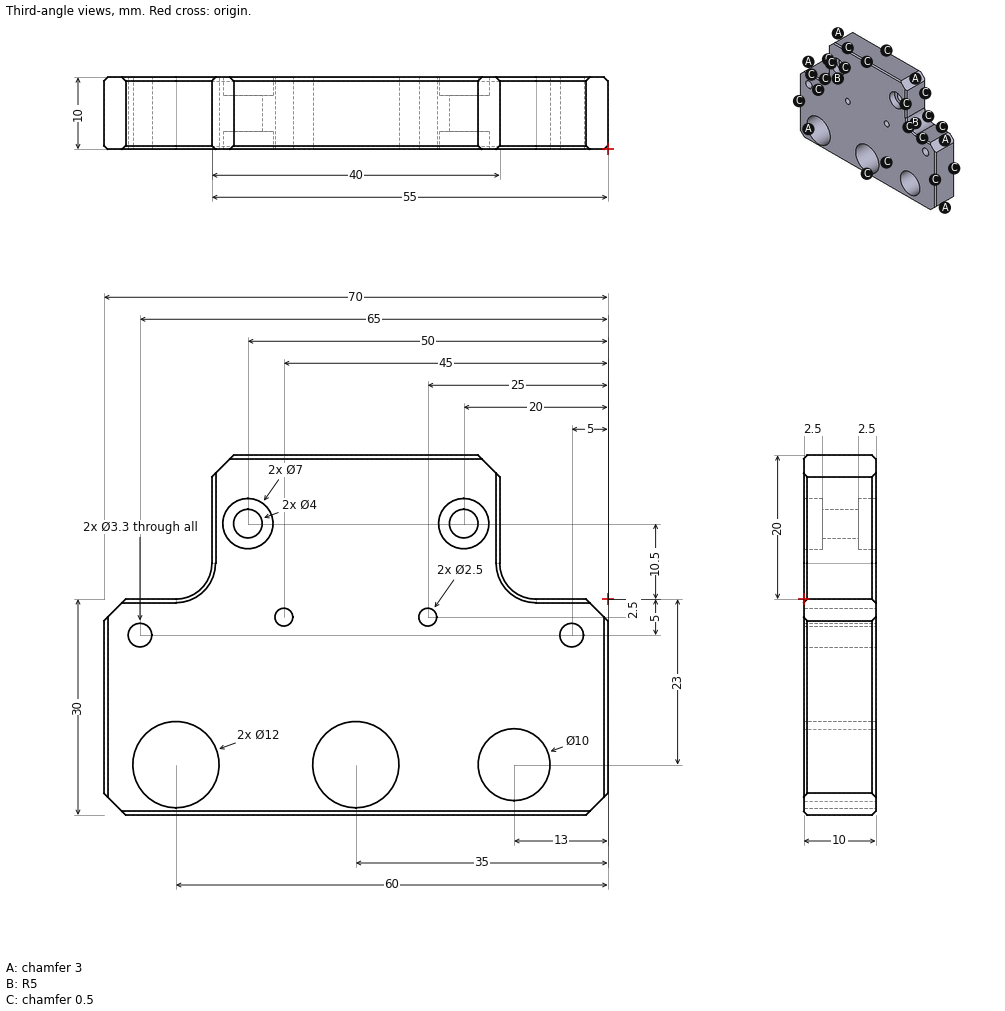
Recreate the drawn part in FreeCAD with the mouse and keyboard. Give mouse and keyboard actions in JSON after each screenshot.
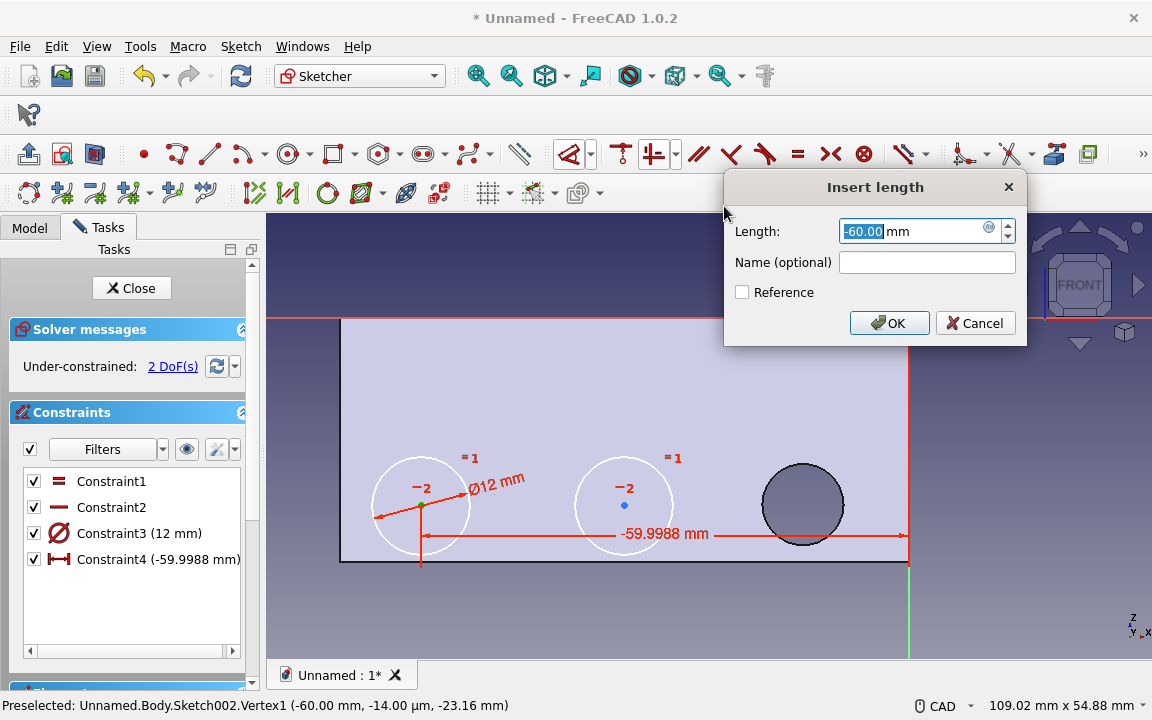
{"action": "type", "text": "-60"}
{"action": "key", "text": "Return"}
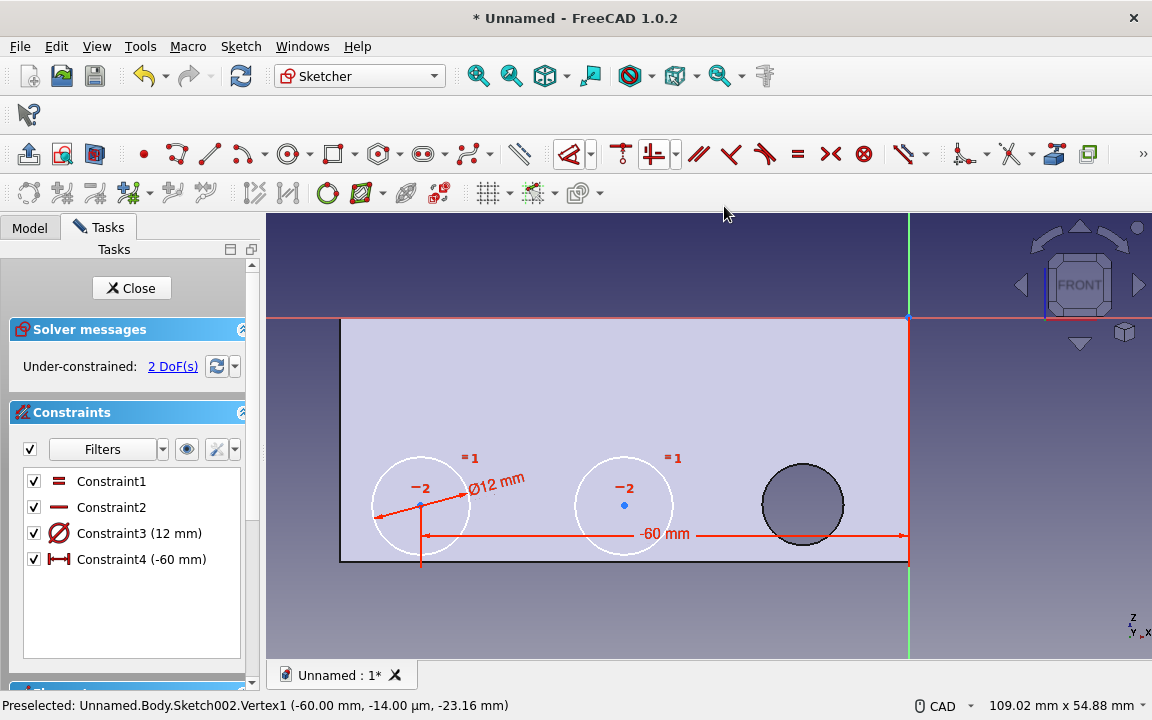
{"action": "left_click", "coordinate": [421, 506]}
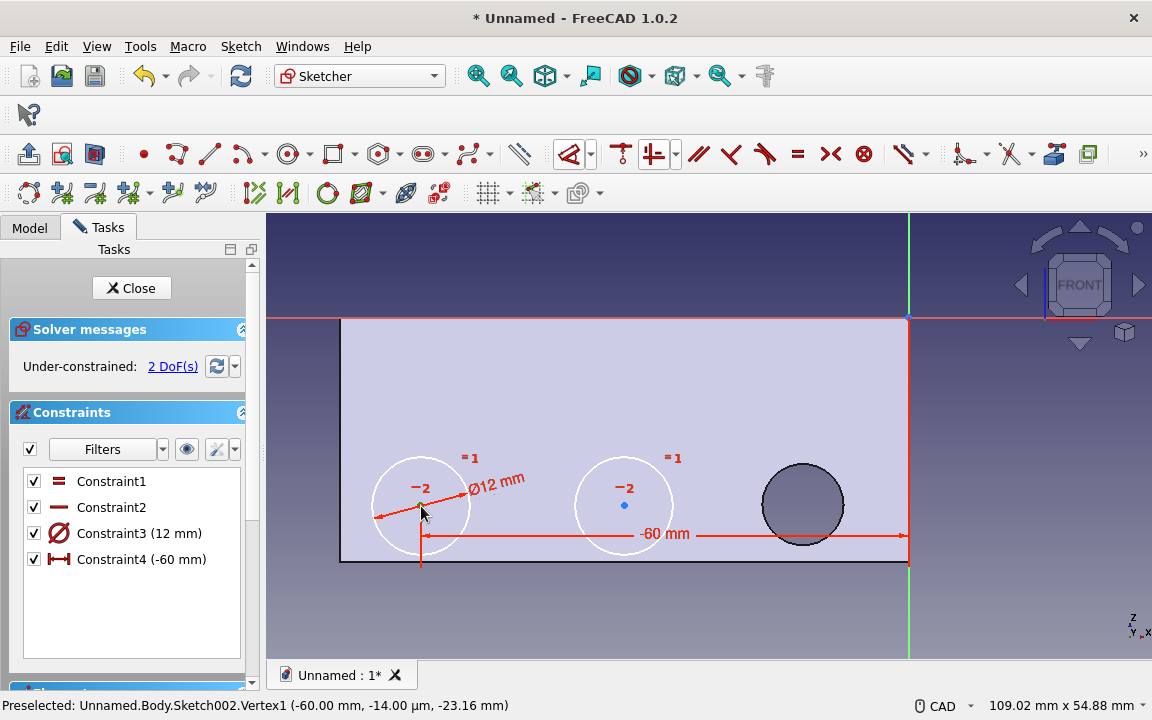
{"action": "left_click", "coordinate": [590, 154]}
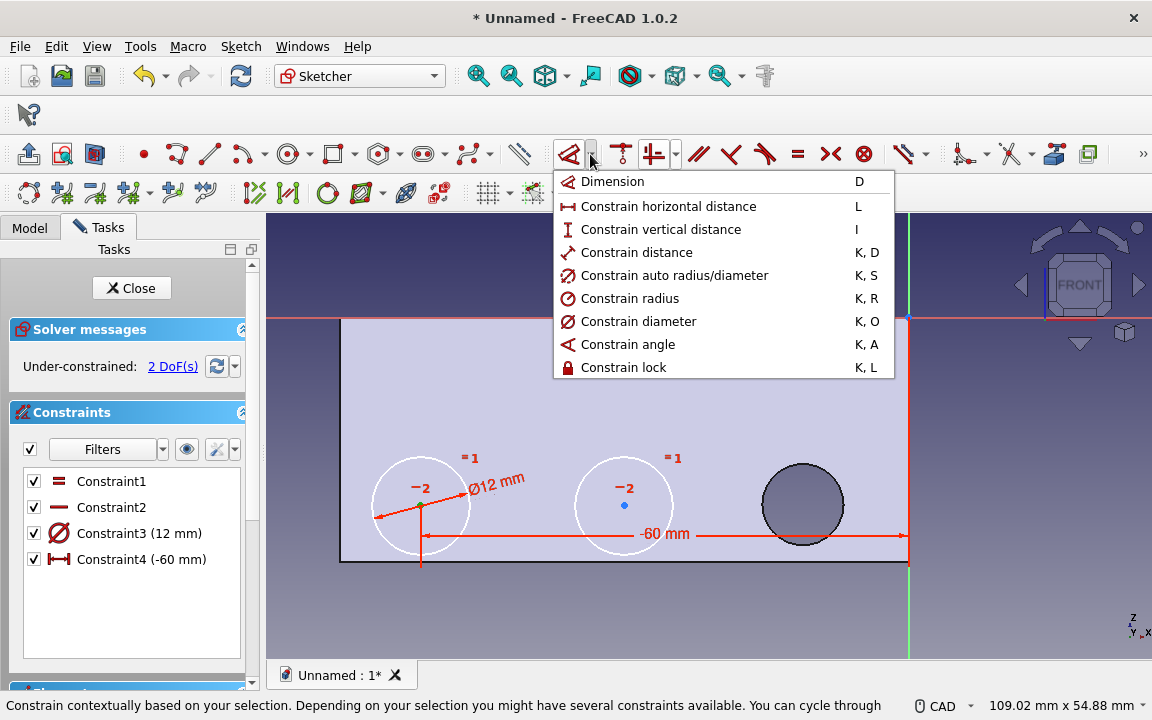
{"action": "left_click", "coordinate": [724, 230]}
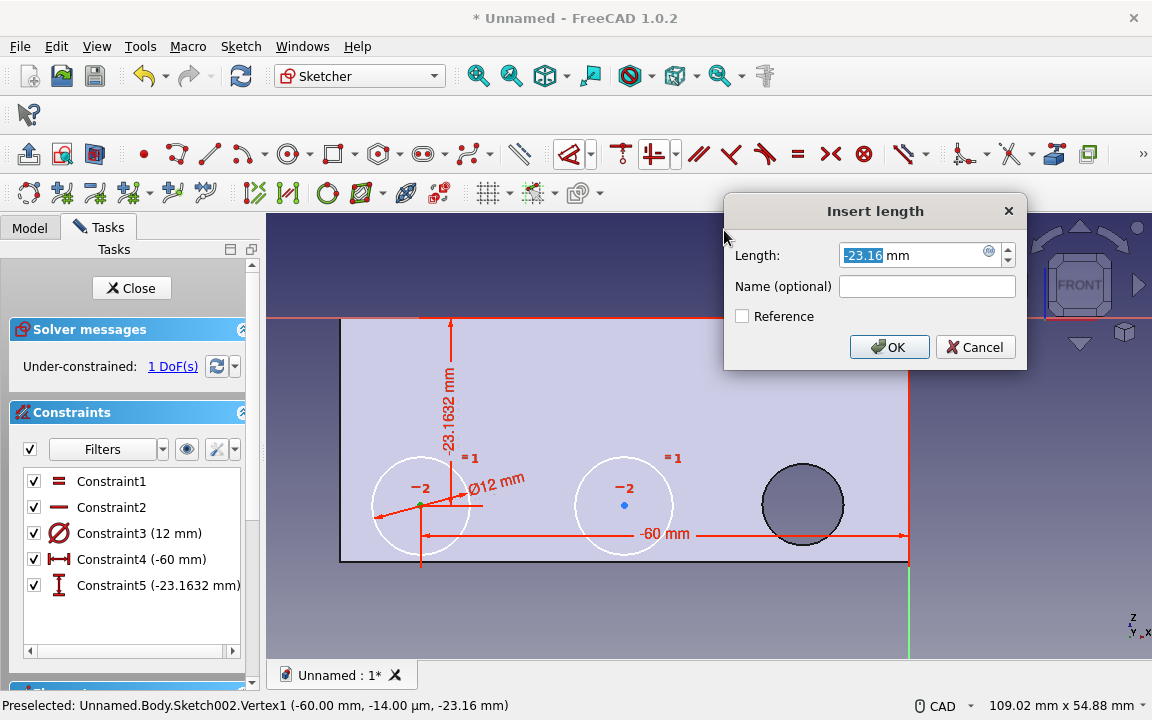
{"action": "type", "text": "-23"}
{"action": "key", "text": "Return"}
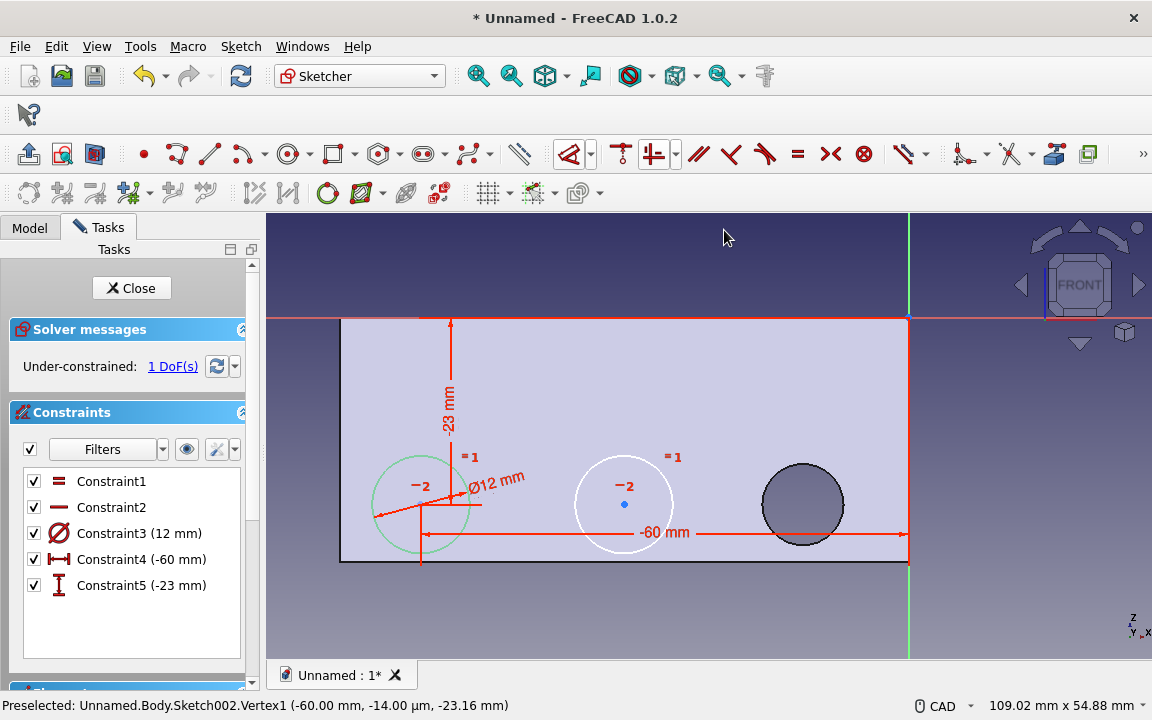
{"action": "left_click", "coordinate": [624, 505]}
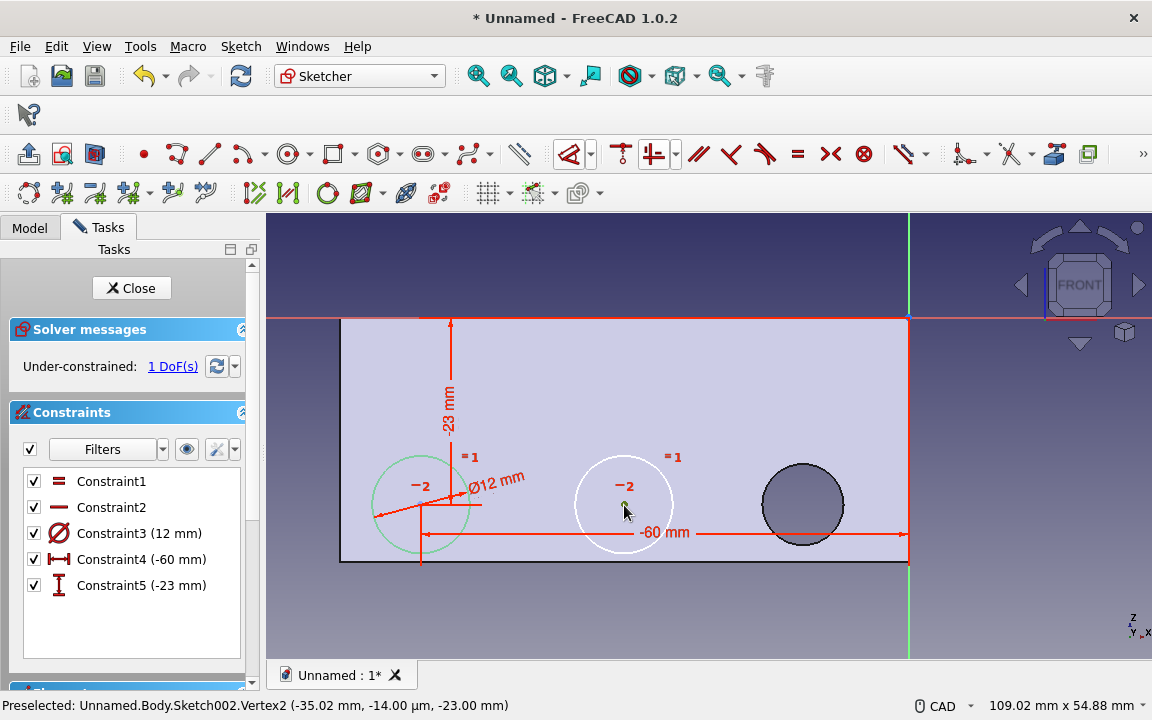
{"action": "key", "text": "l"}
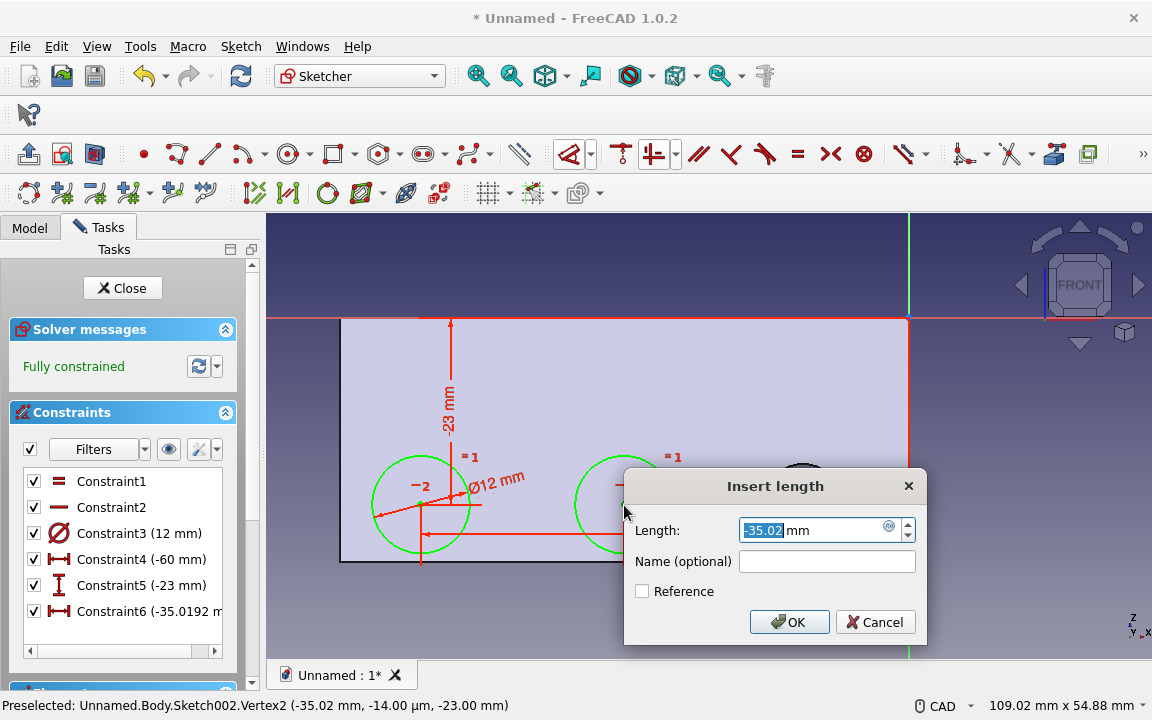
{"action": "type", "text": "-35"}
{"action": "key", "text": "Return"}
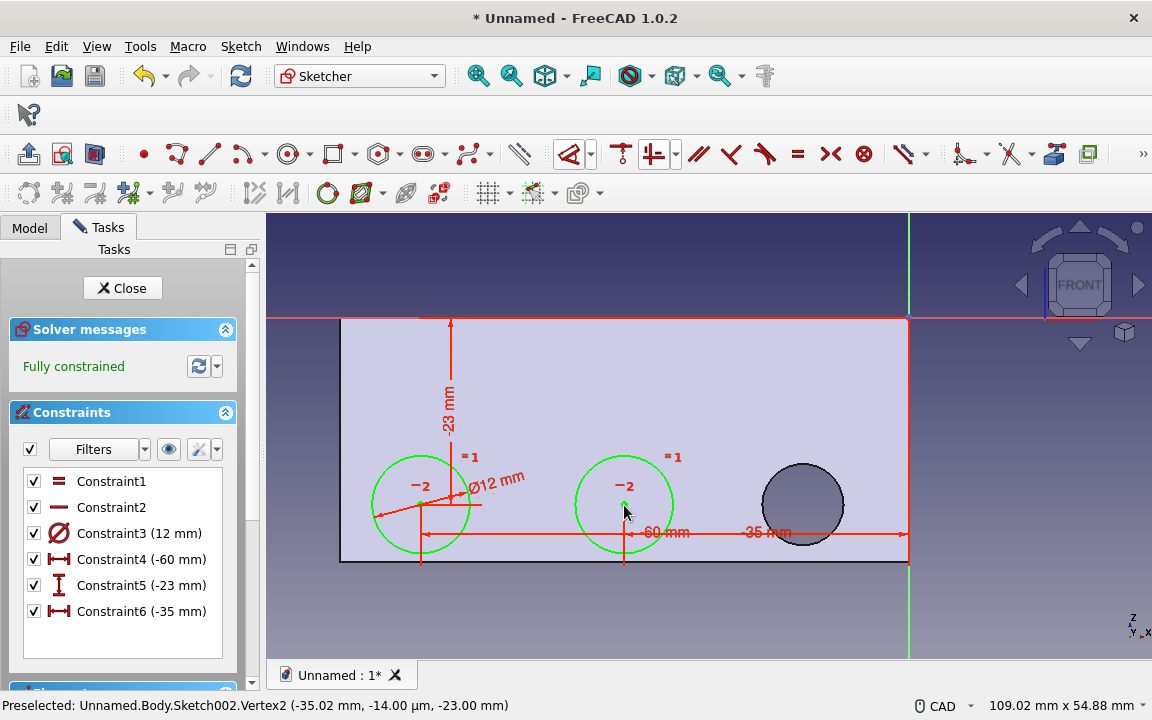
{"action": "left_click", "coordinate": [123, 288]}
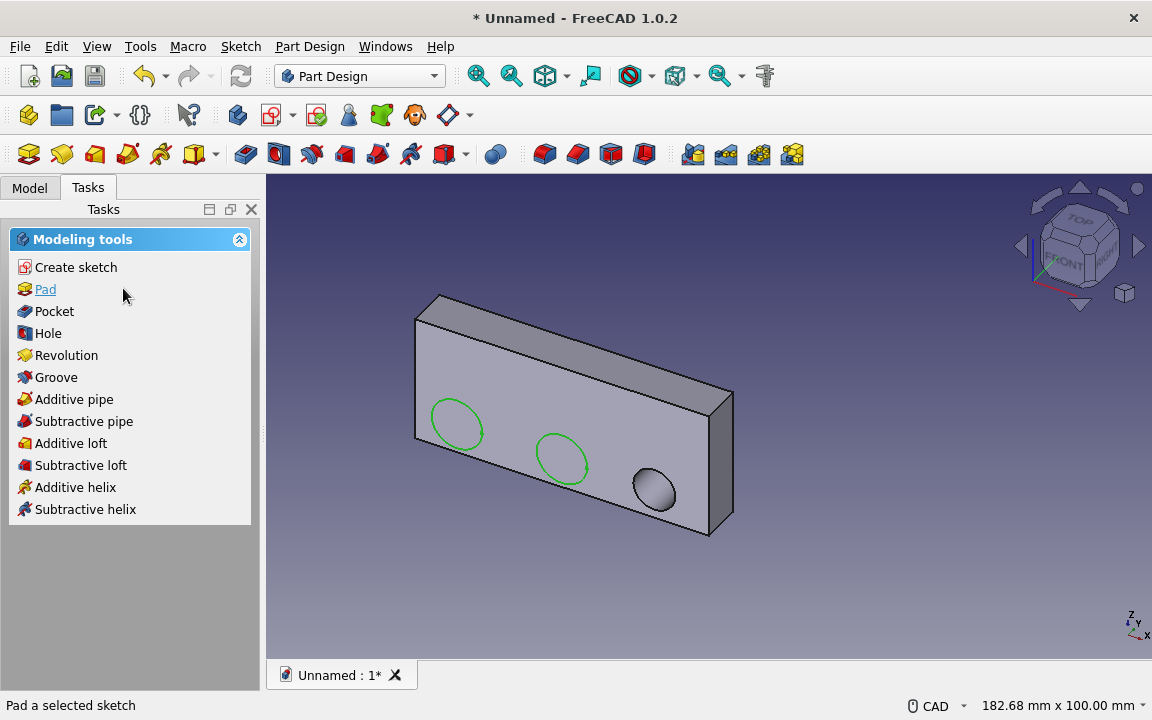
{"action": "left_click", "coordinate": [246, 154]}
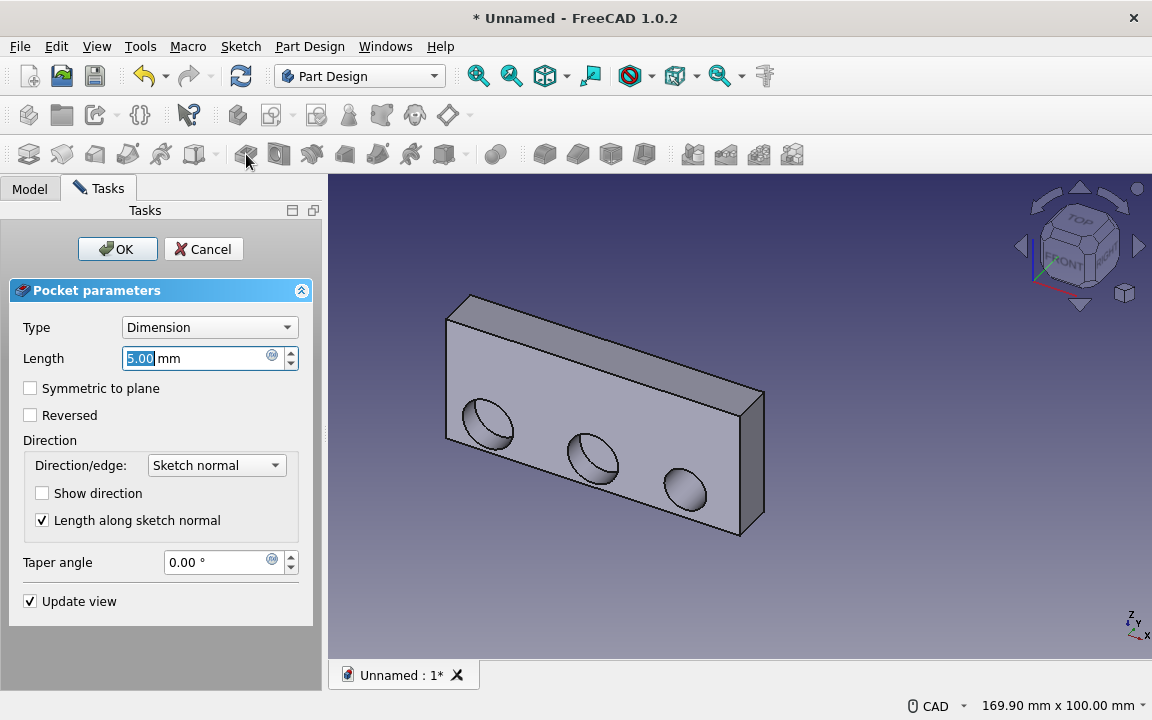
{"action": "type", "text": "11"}
{"action": "key", "text": "Tab"}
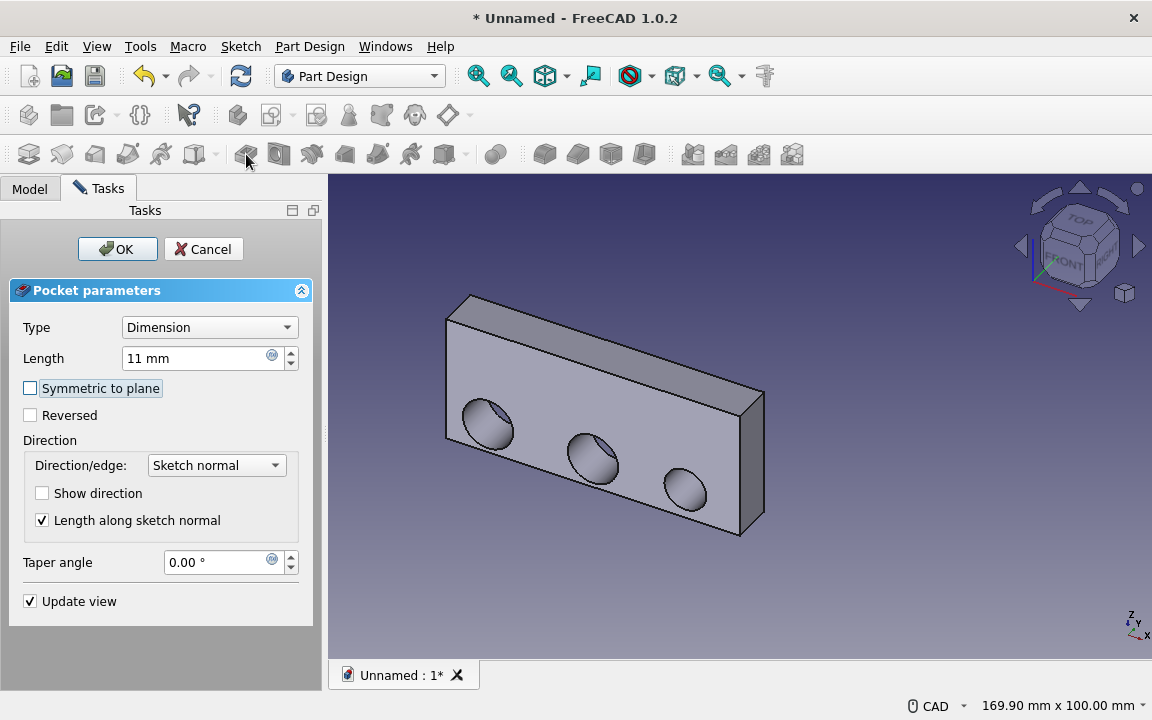
{"action": "left_click", "coordinate": [118, 249]}